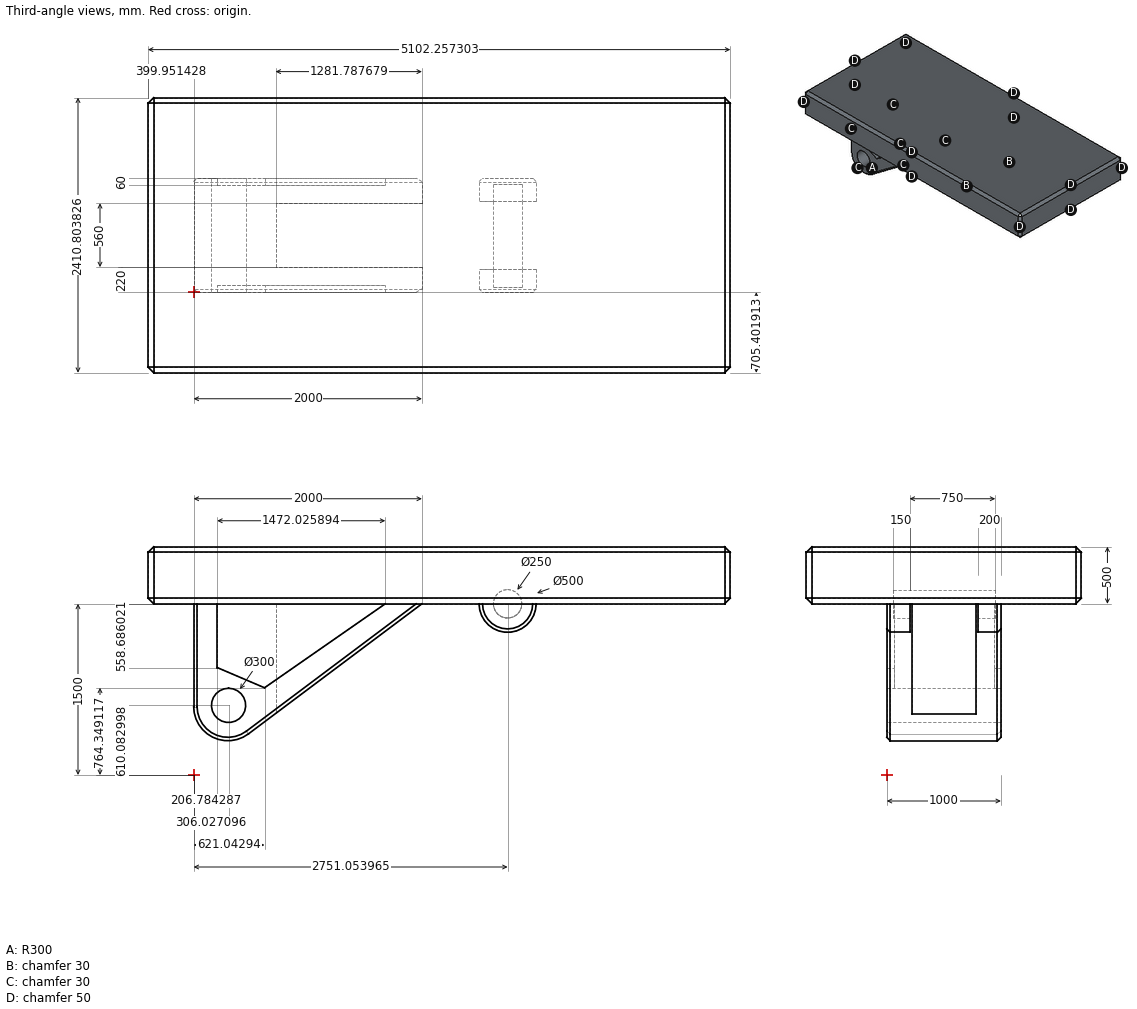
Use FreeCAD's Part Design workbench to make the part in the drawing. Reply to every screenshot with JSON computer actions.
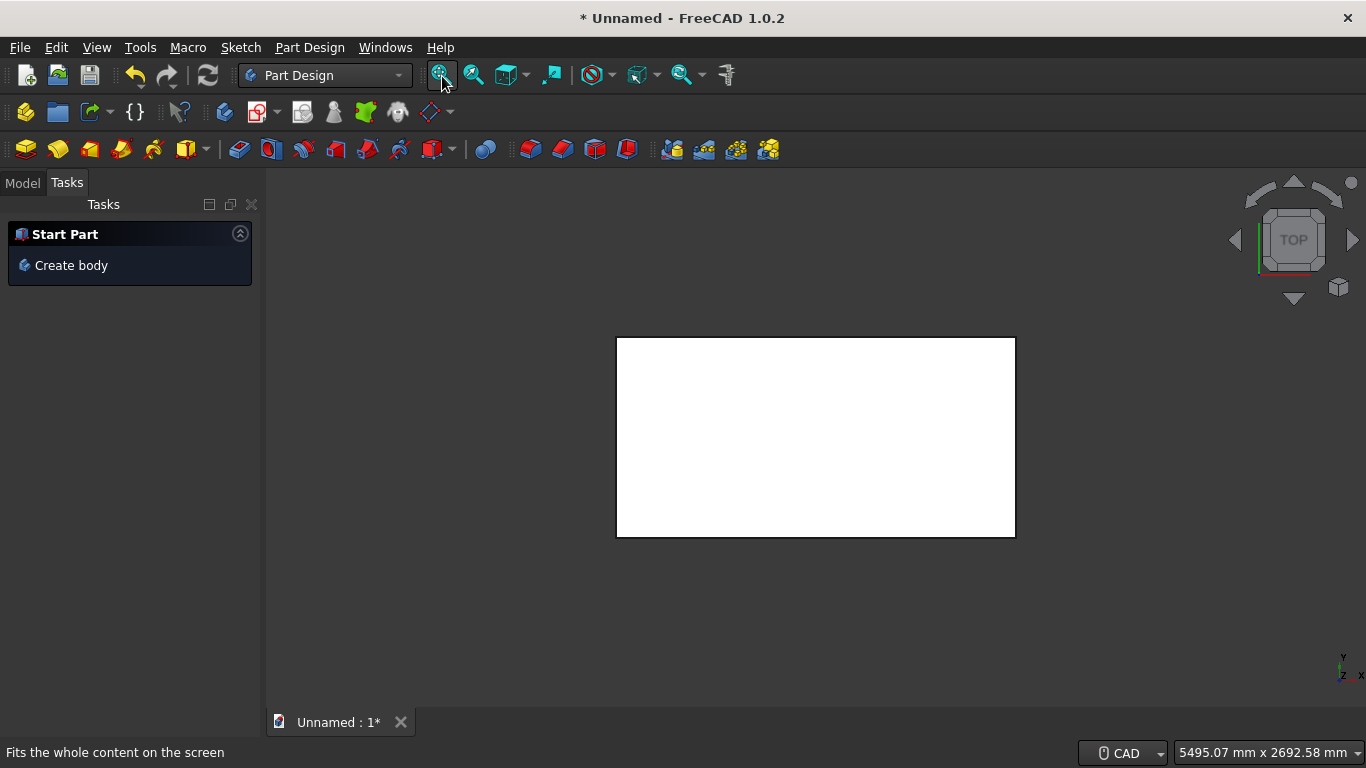
{"action": "left_click", "coordinate": [442, 76]}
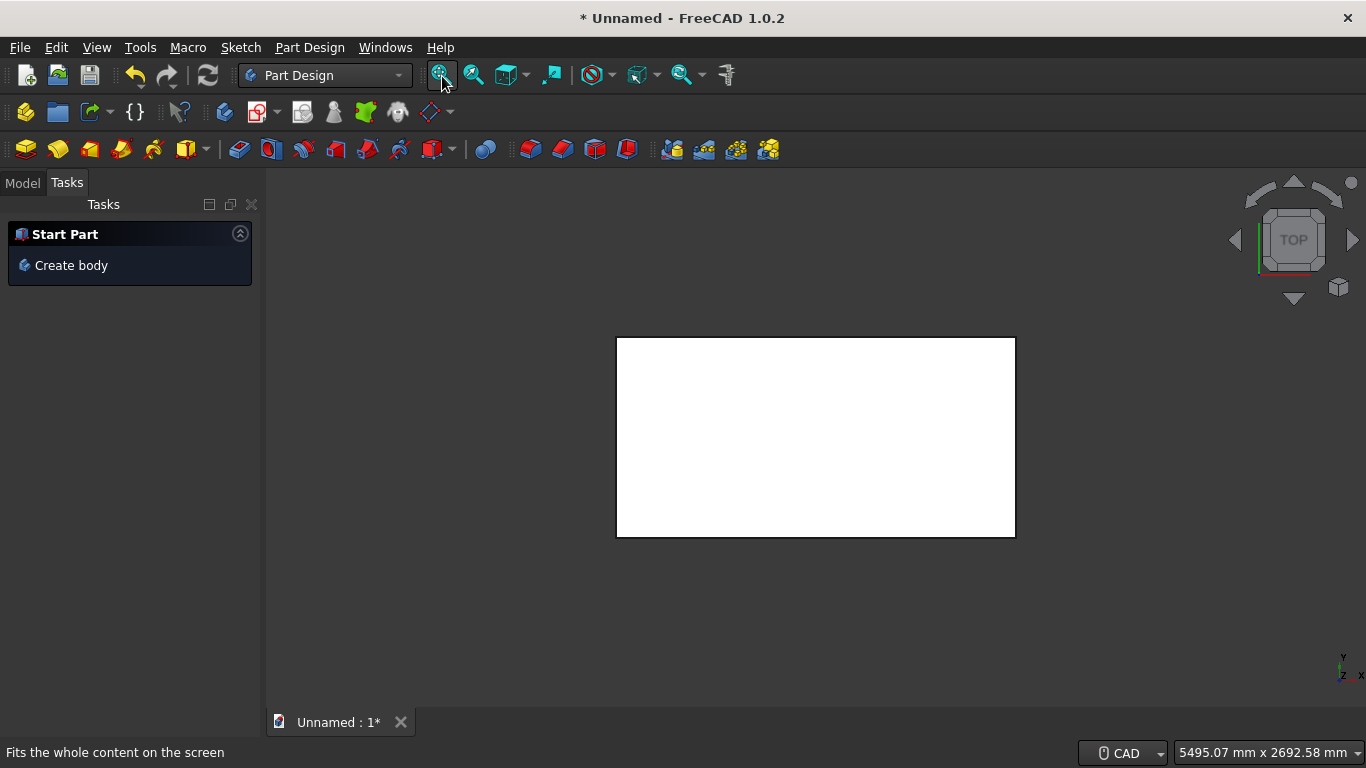
{"action": "key", "text": "1"}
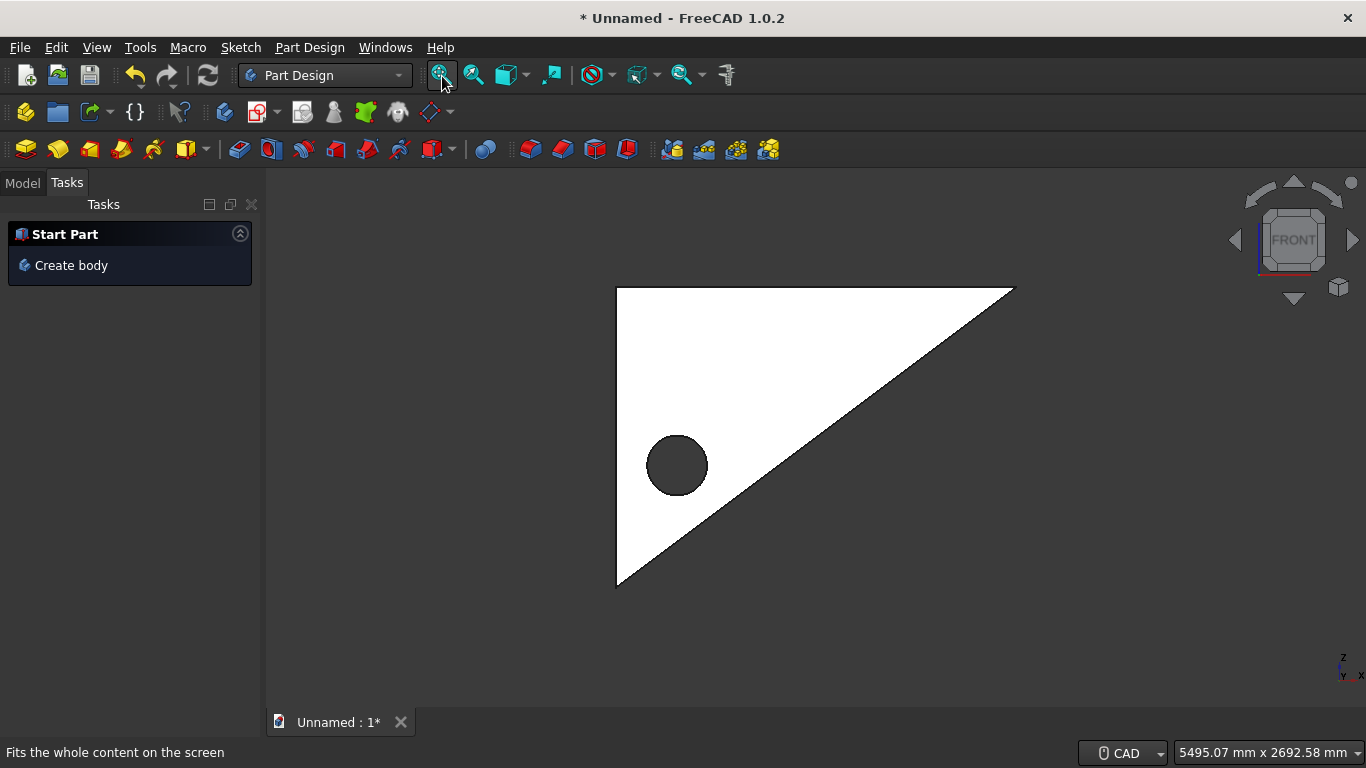
{"action": "key", "text": "3"}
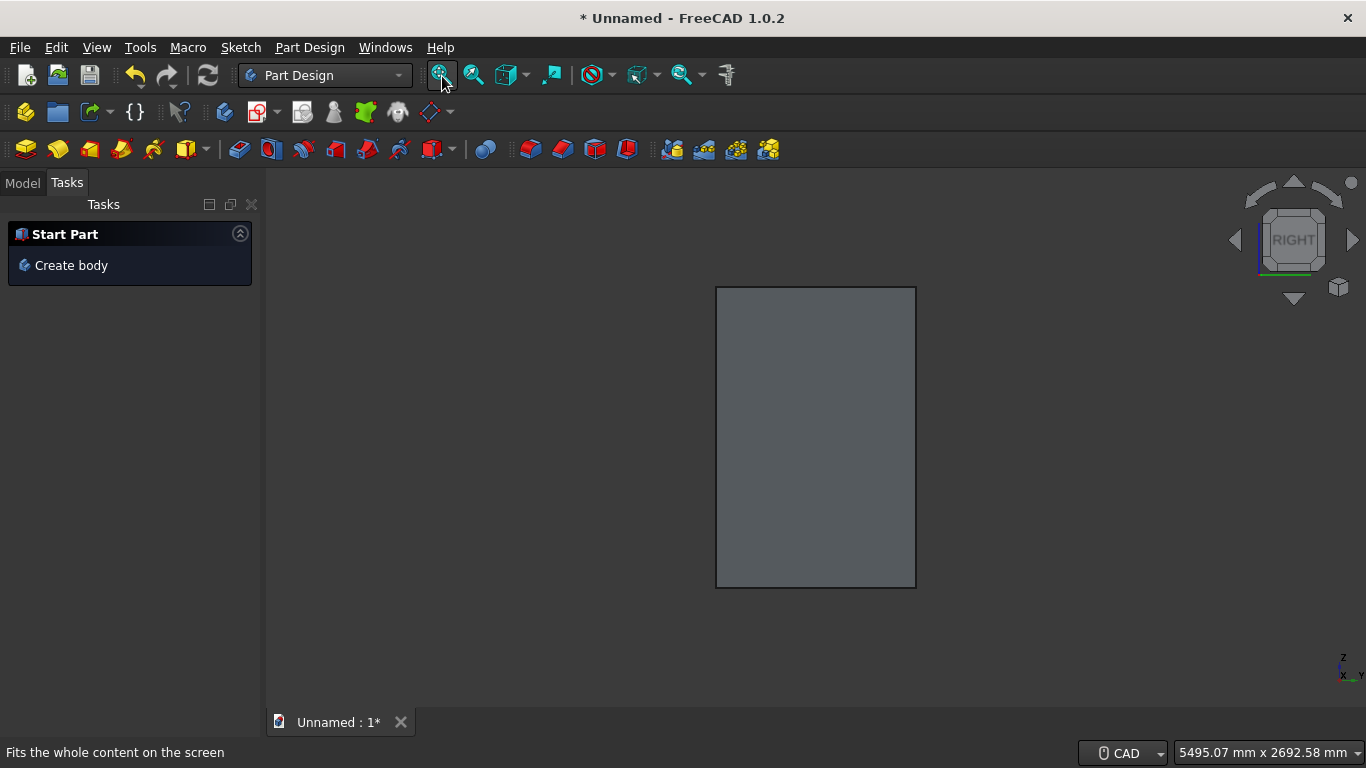
{"action": "key", "text": "5"}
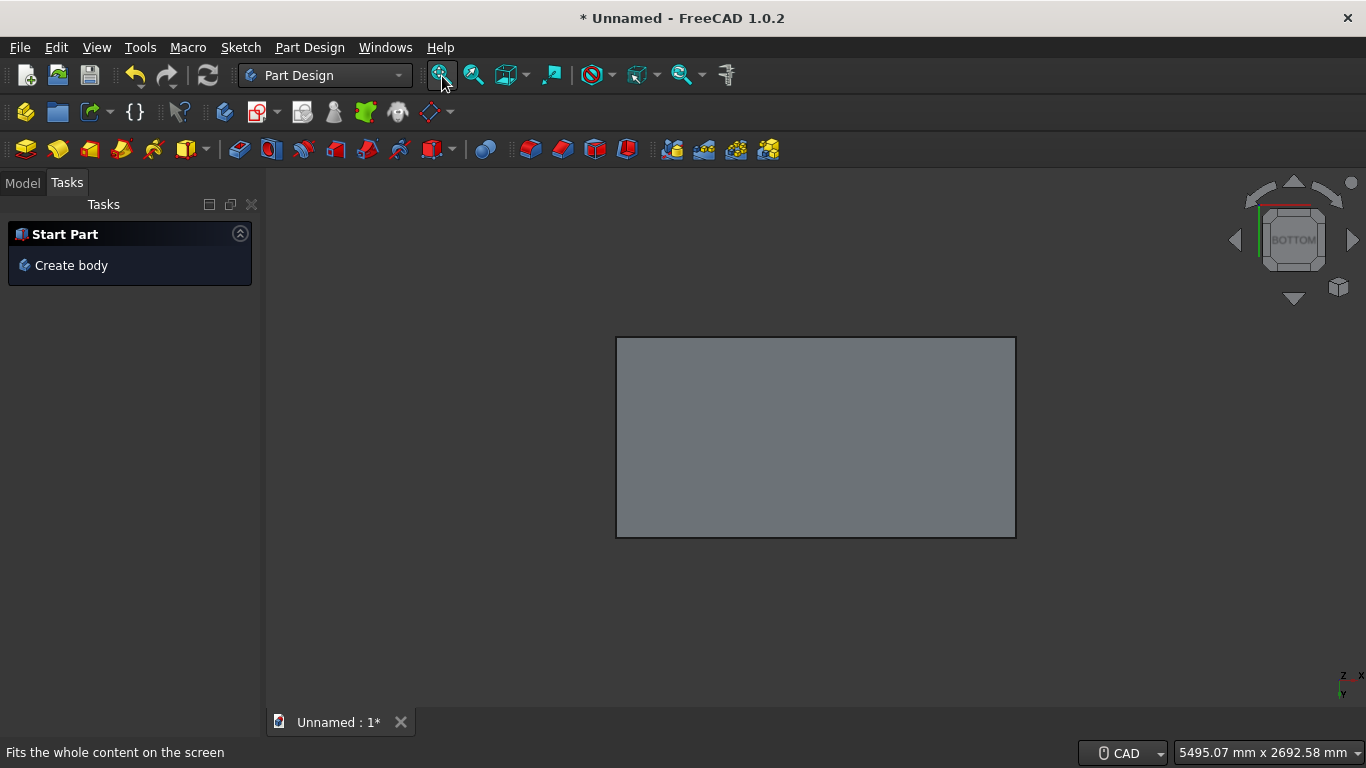
{"action": "left_click", "coordinate": [442, 76]}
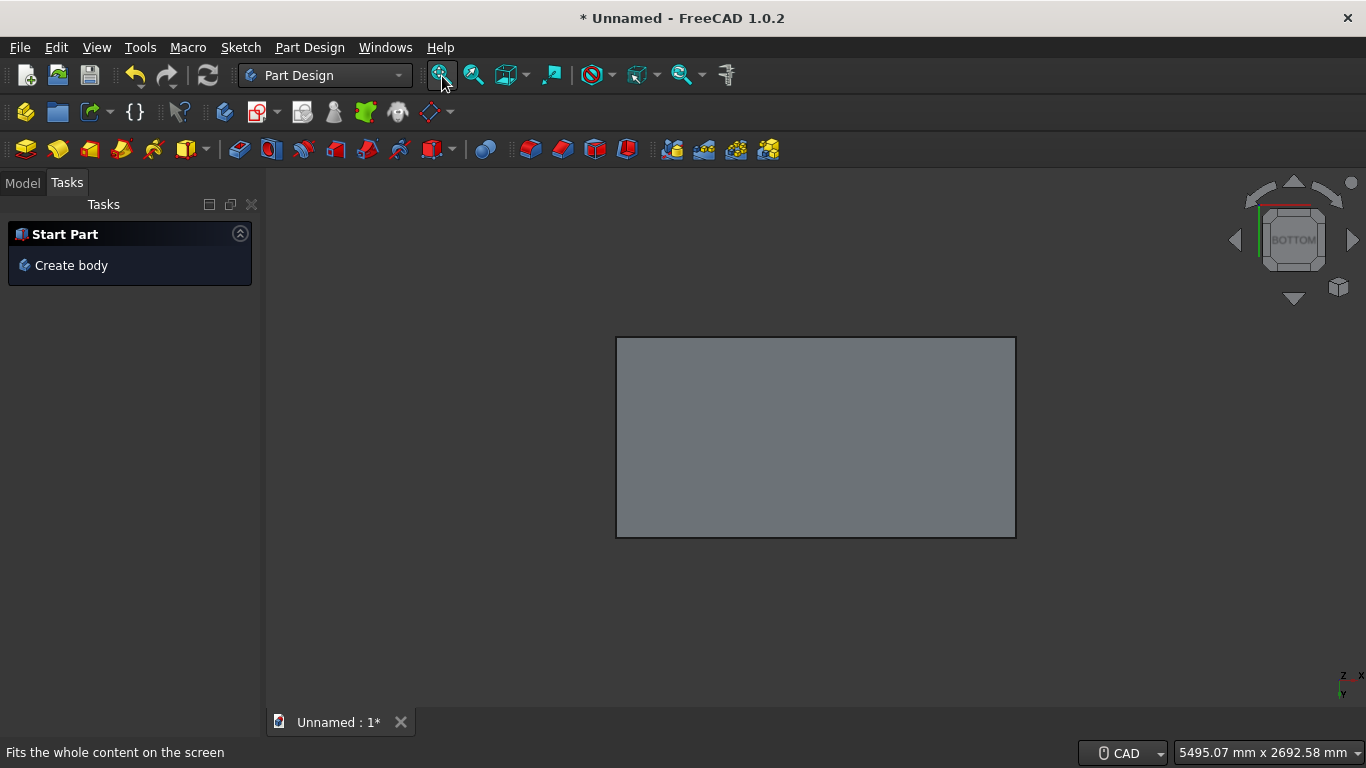
{"action": "left_click", "coordinate": [616, 436]}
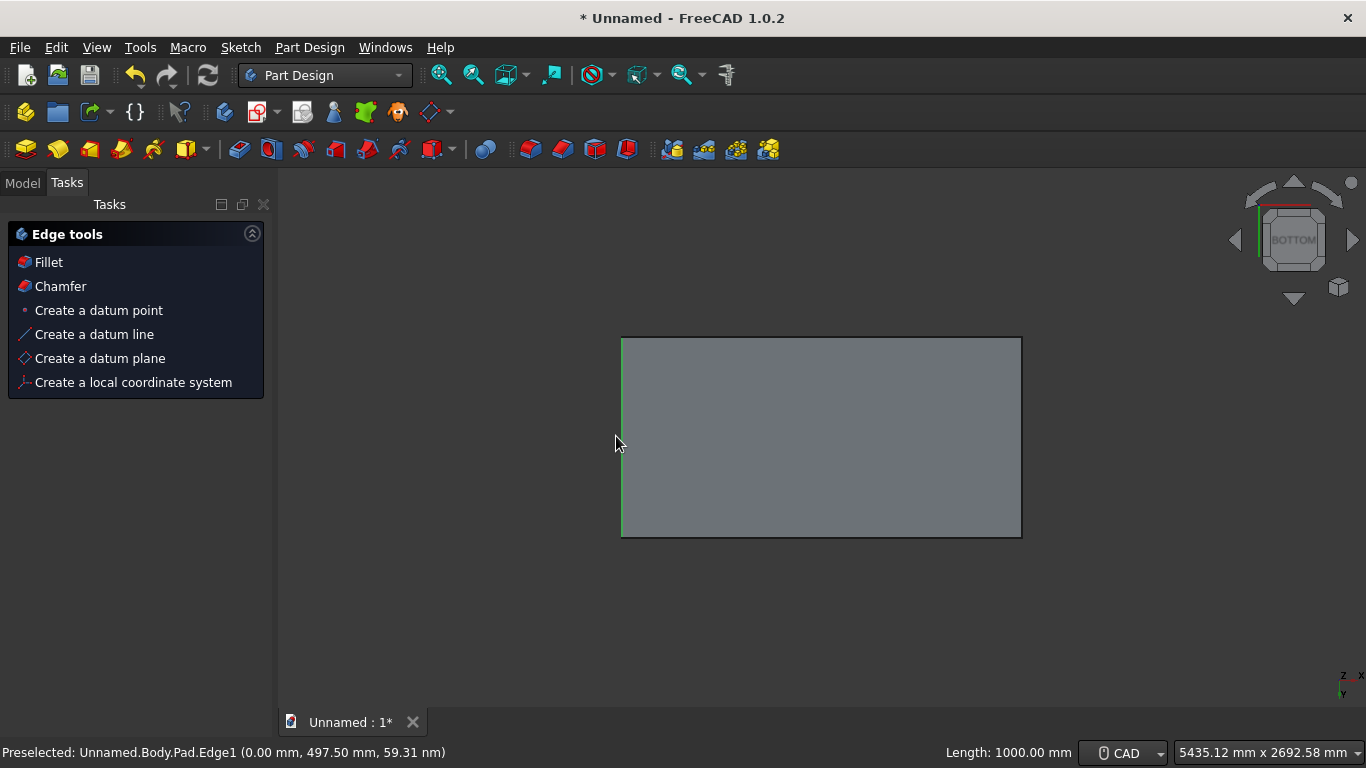
{"action": "left_click", "coordinate": [532, 150]}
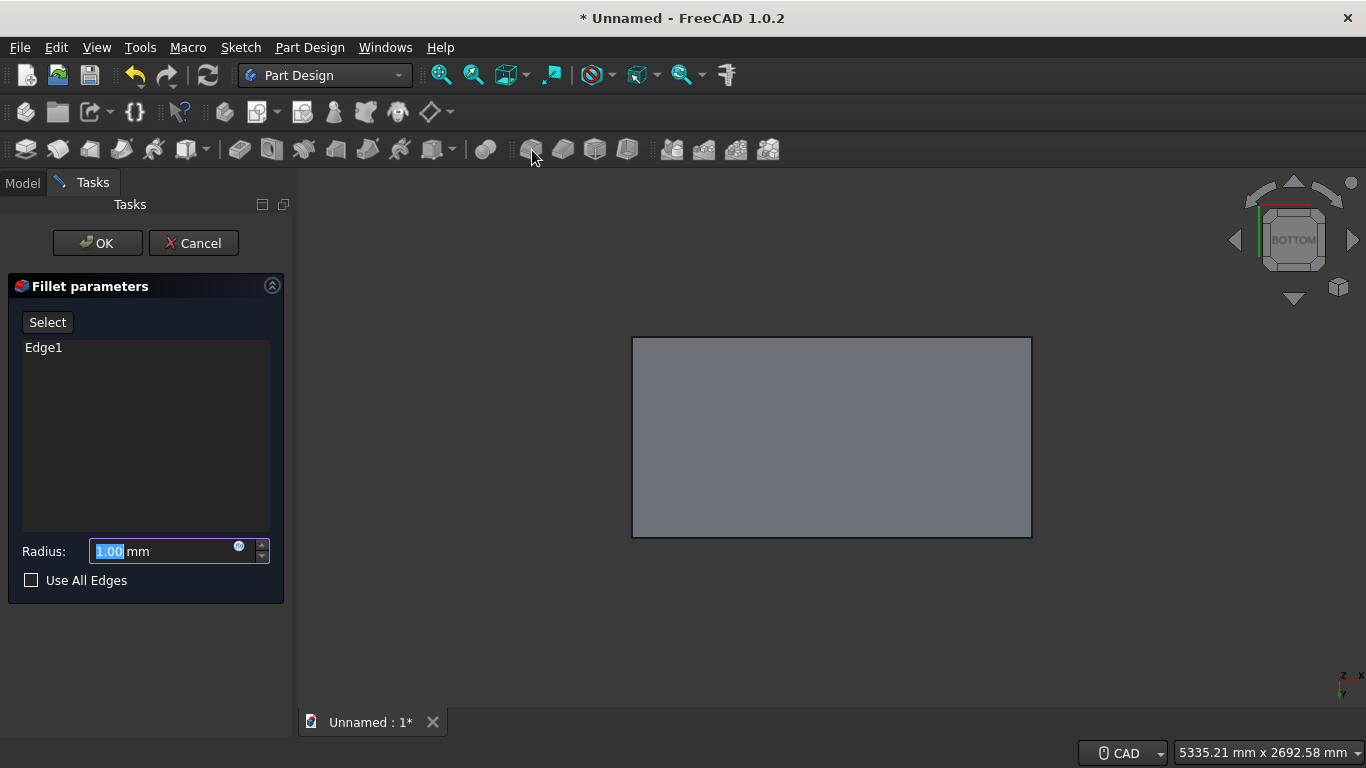
{"action": "type", "text": "300"}
{"action": "key", "text": "Tab"}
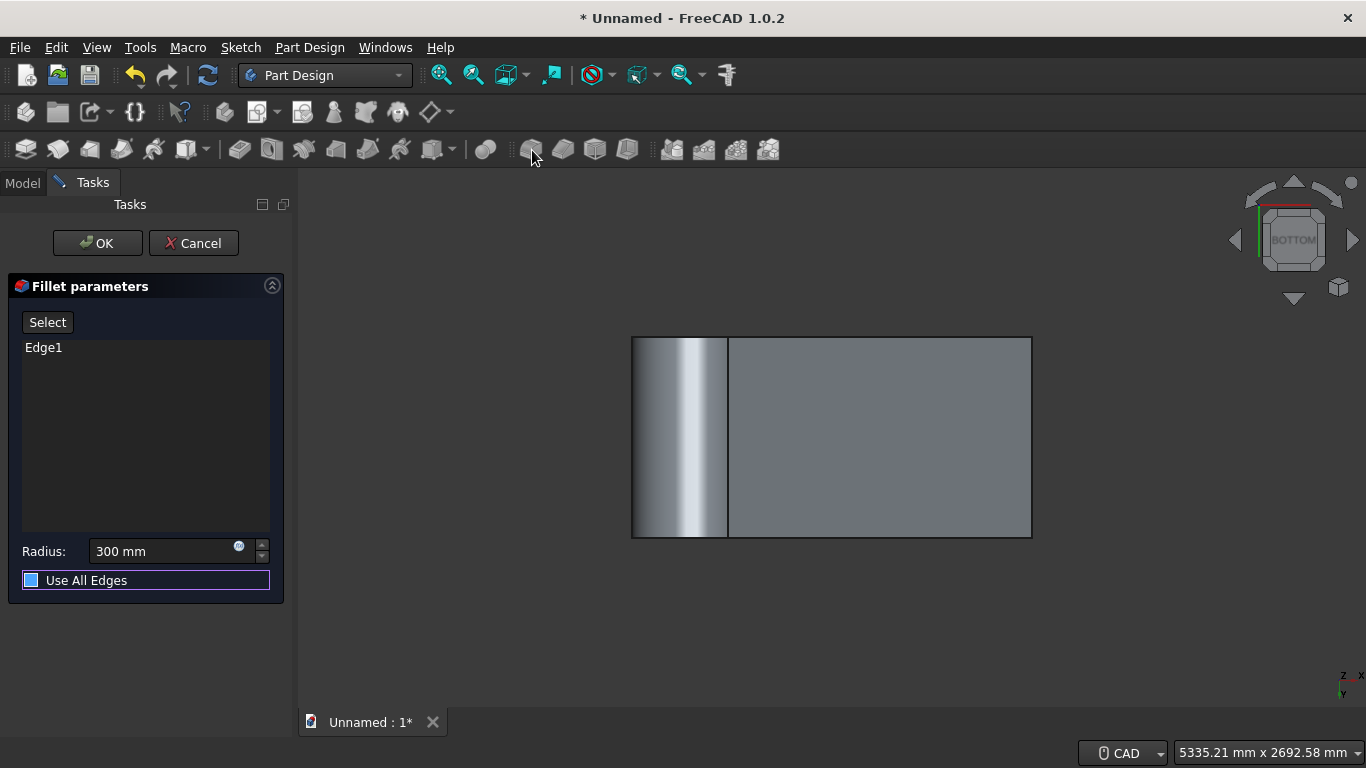
{"action": "left_click", "coordinate": [98, 243]}